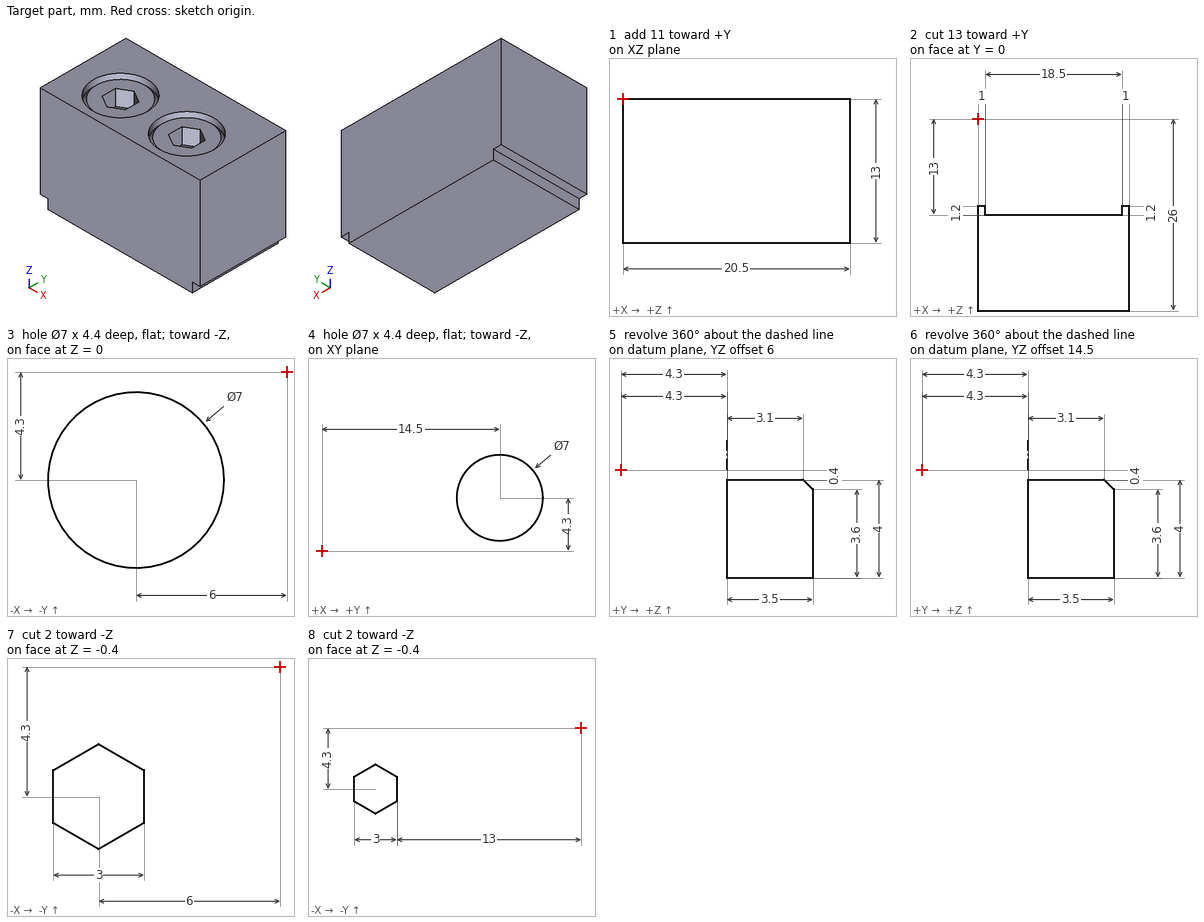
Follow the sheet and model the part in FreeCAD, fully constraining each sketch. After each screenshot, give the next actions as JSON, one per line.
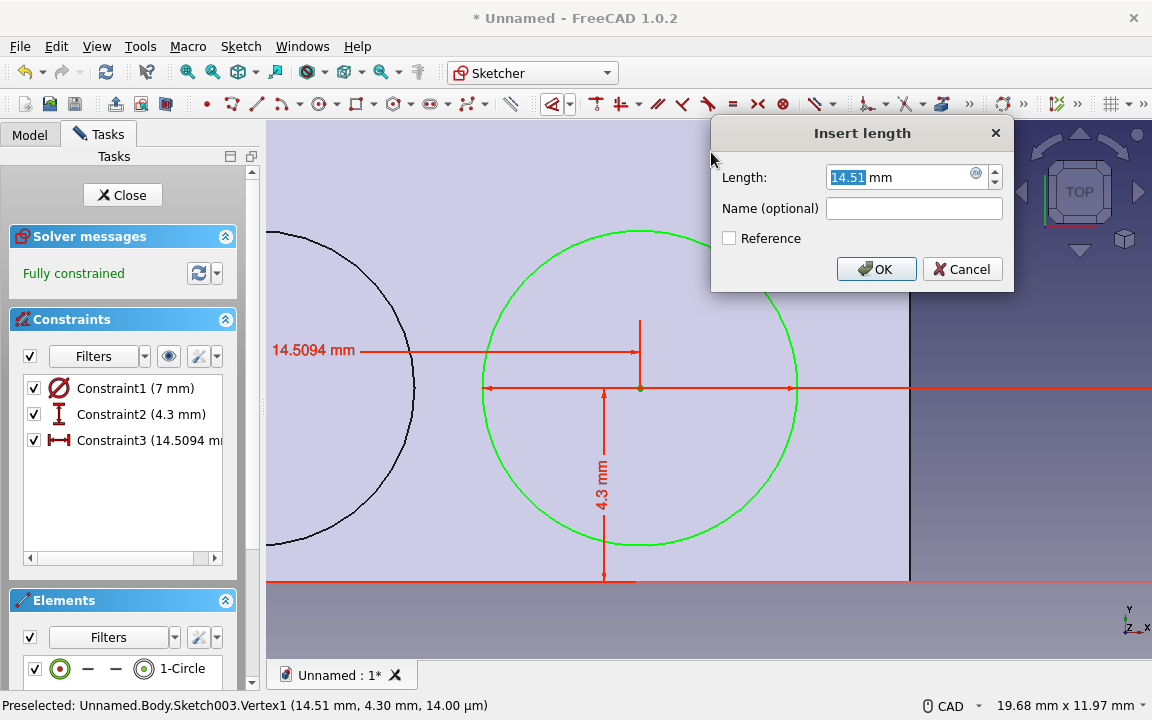
{"action": "type", "text": "14.5"}
{"action": "key", "text": "Return"}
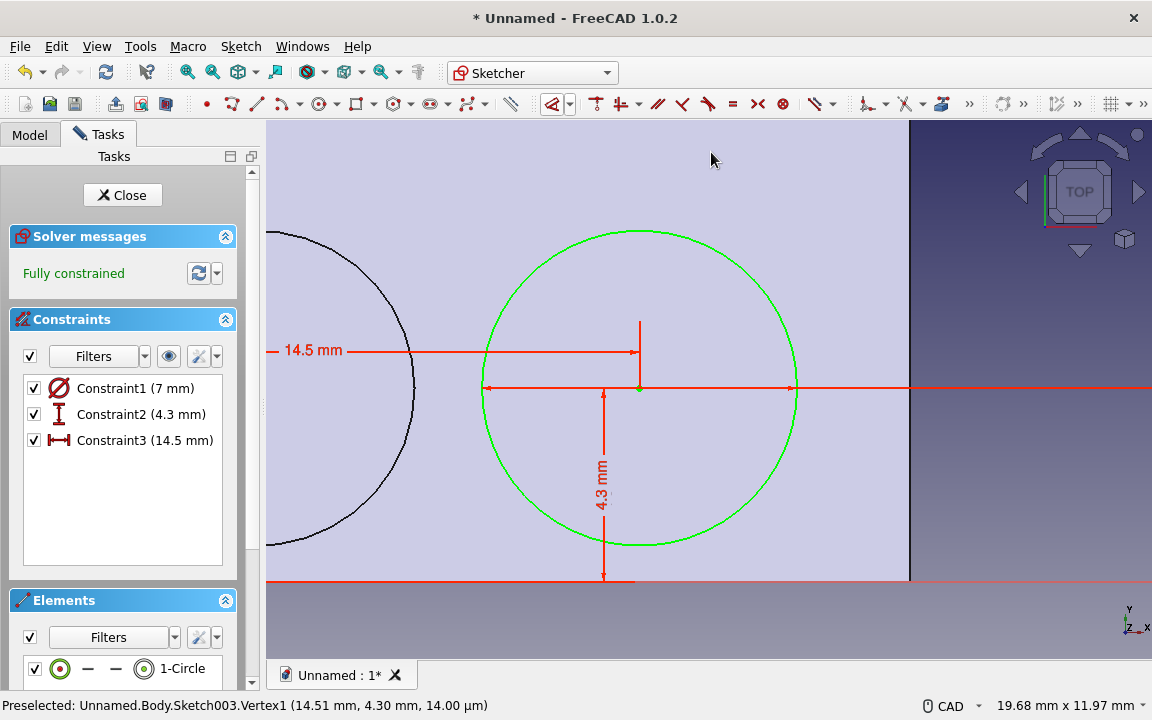
{"action": "left_click", "coordinate": [123, 195]}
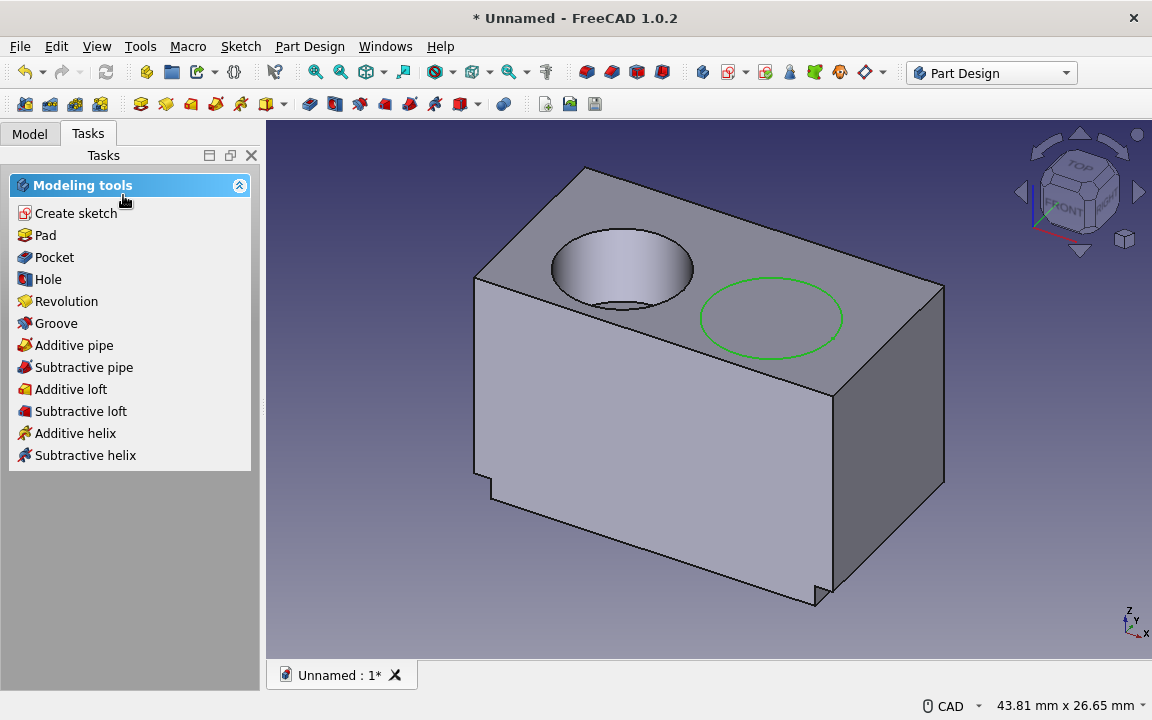
{"action": "left_click", "coordinate": [335, 104]}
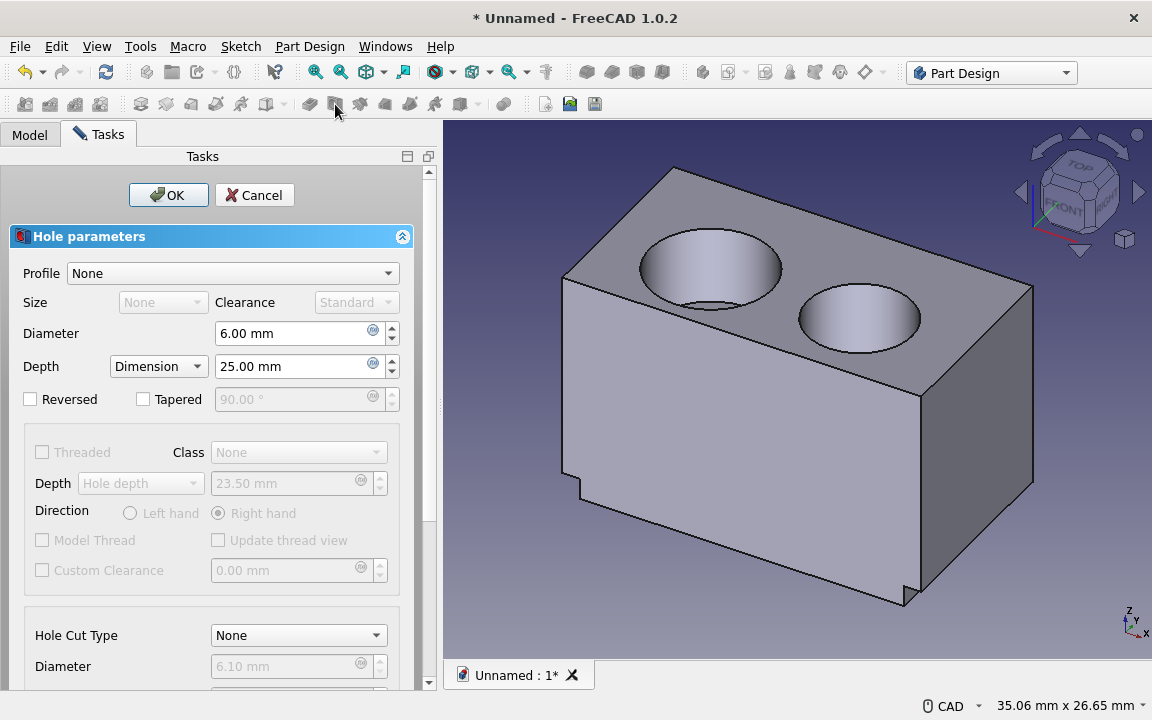
{"action": "triple_click", "coordinate": [300, 334]}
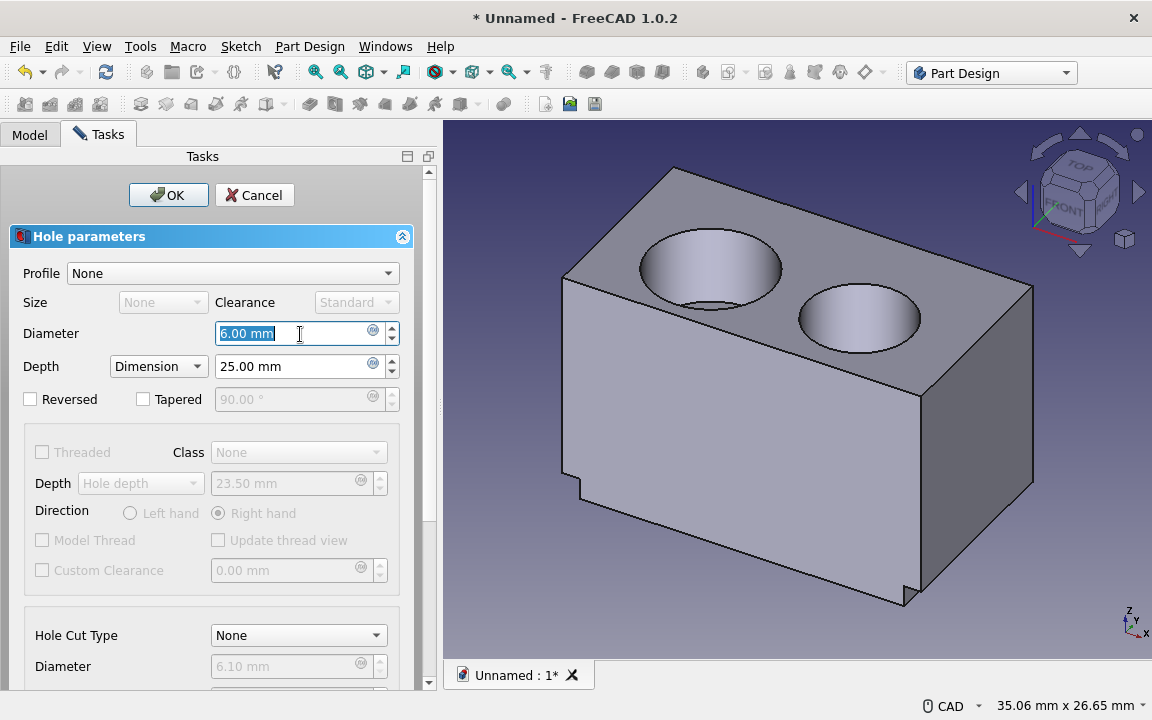
{"action": "type", "text": "7"}
{"action": "key", "text": "Tab"}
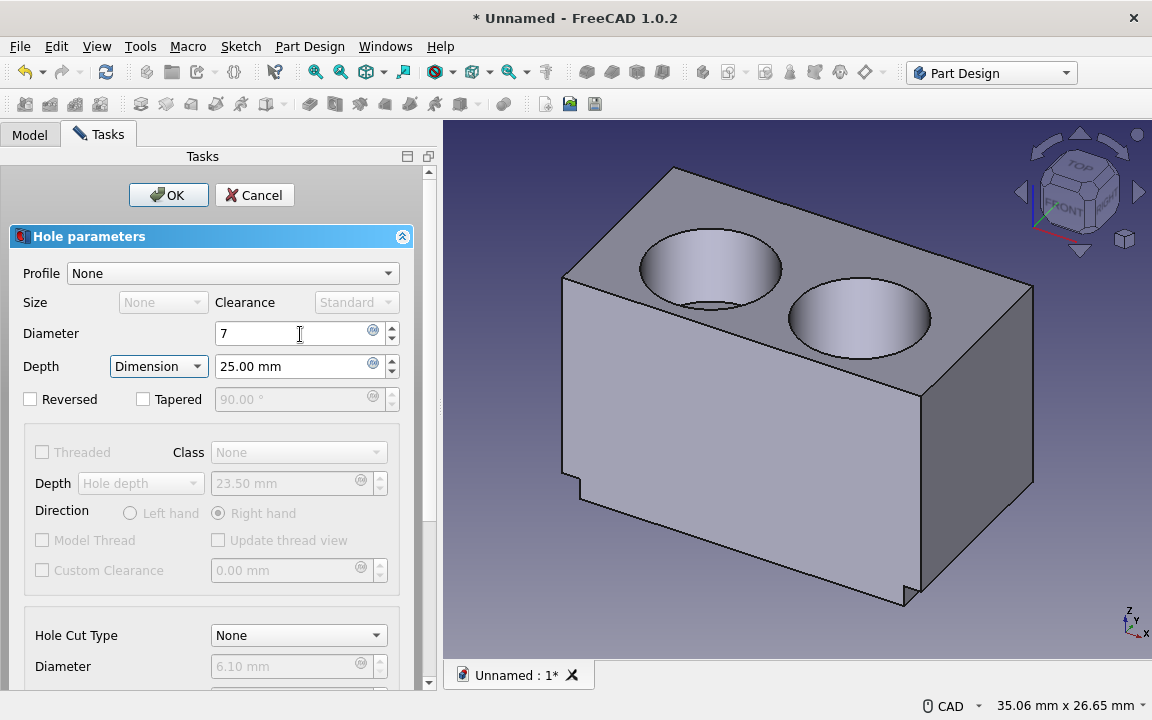
{"action": "triple_click", "coordinate": [300, 366]}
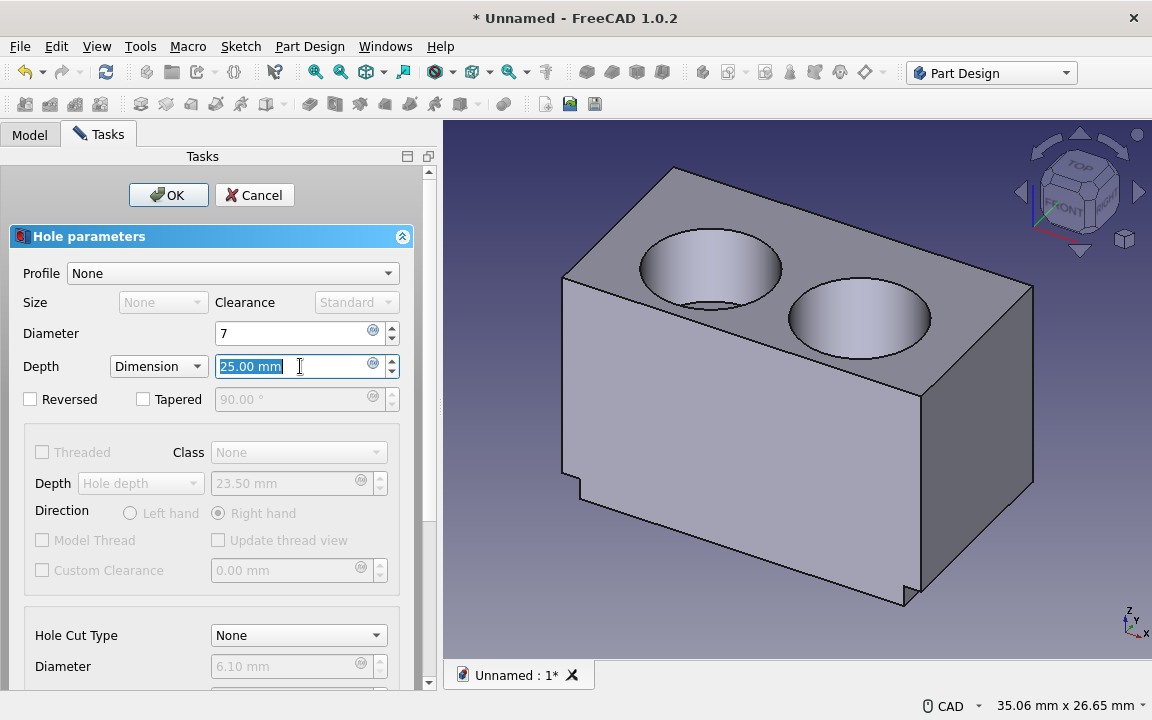
{"action": "type", "text": "4.4"}
{"action": "key", "text": "Tab"}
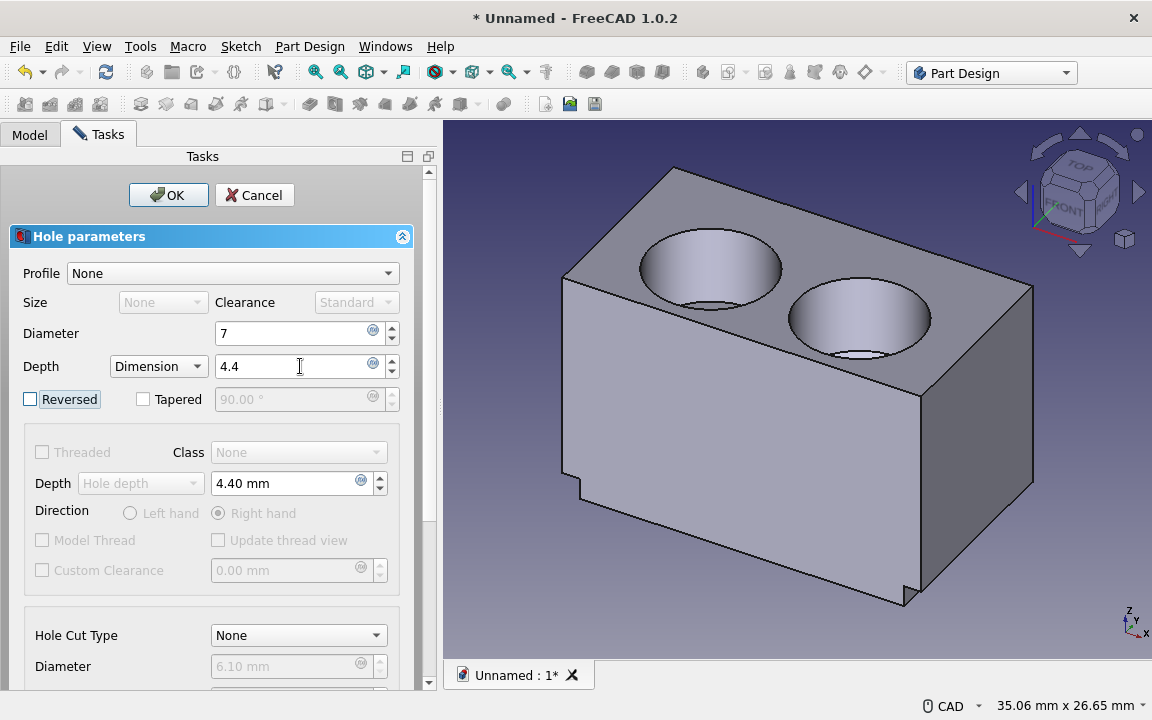
{"action": "scroll", "coordinate": [429, 428], "scroll_direction": "down", "scroll_amount": 4}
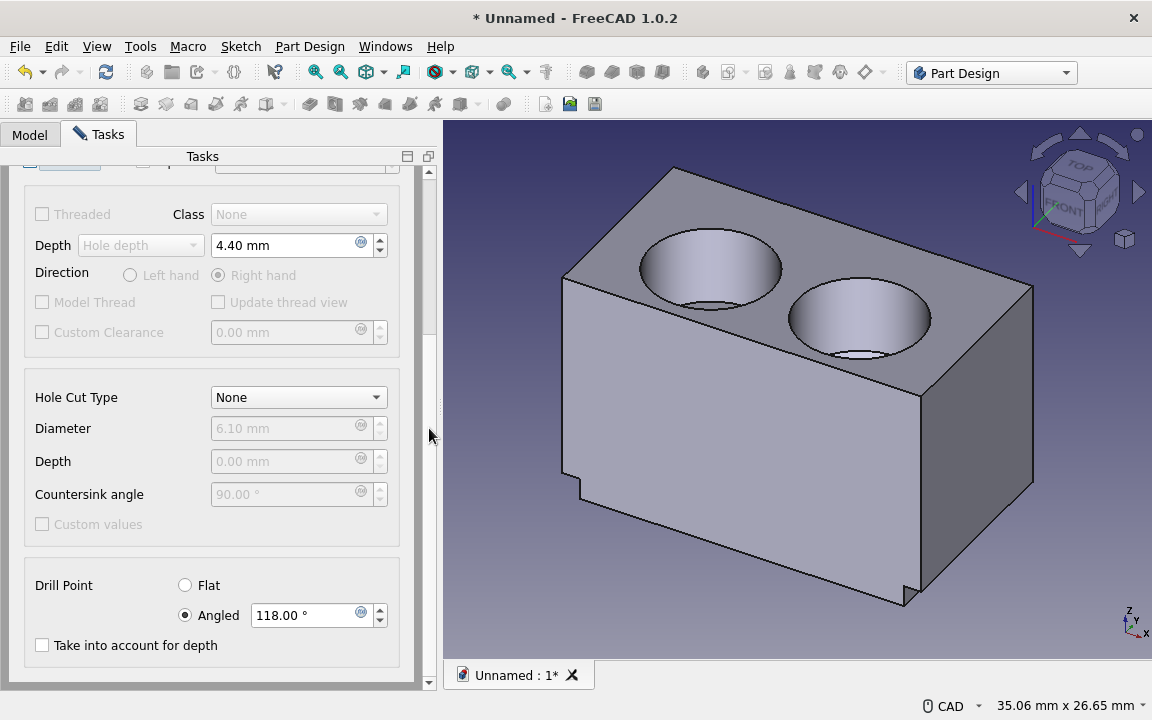
{"action": "left_click", "coordinate": [186, 583]}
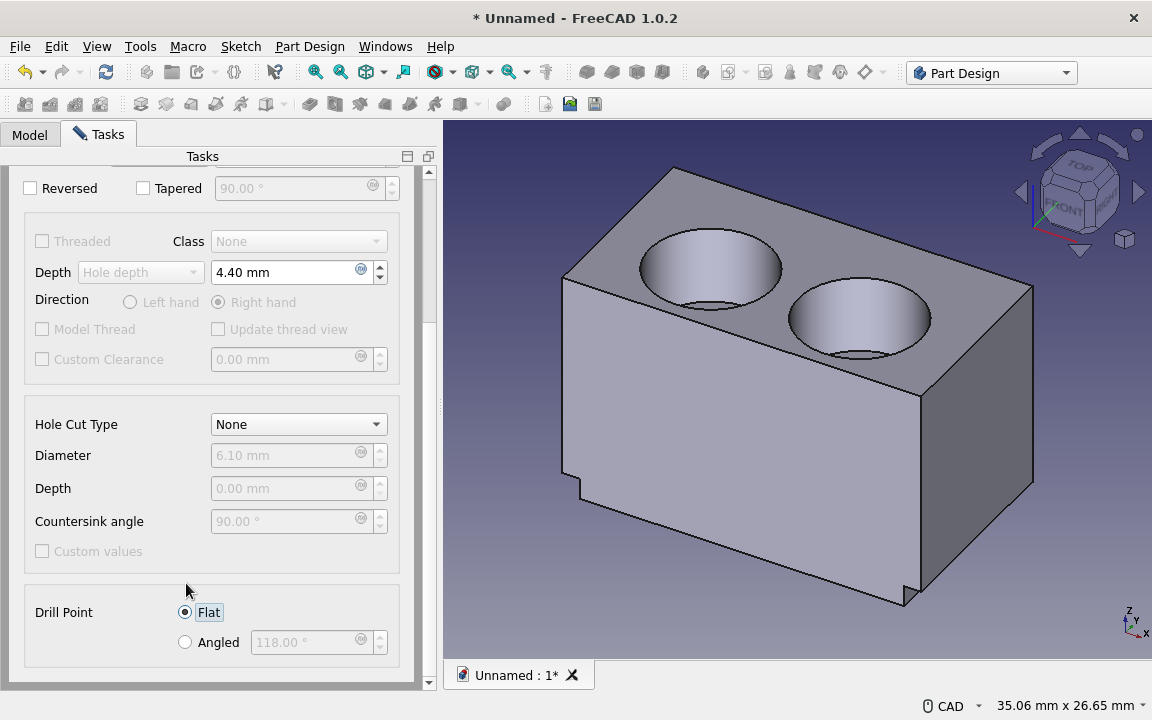
{"action": "scroll", "coordinate": [429, 428], "scroll_direction": "up", "scroll_amount": 5}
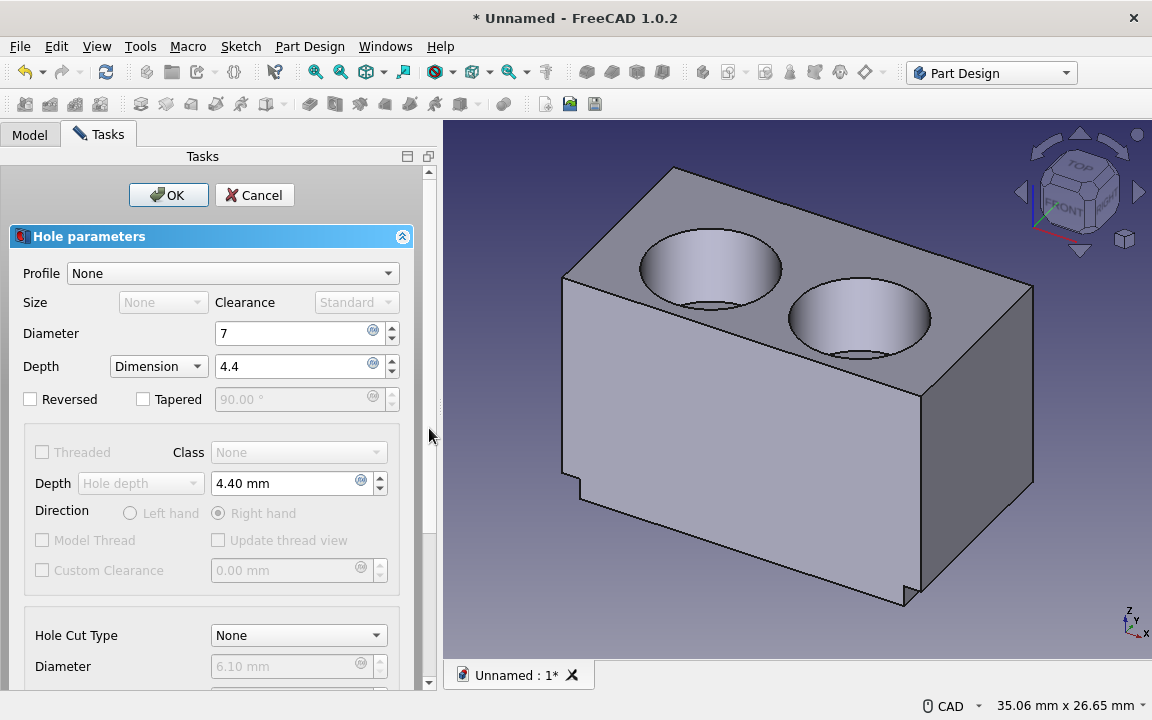
{"action": "left_click", "coordinate": [169, 195]}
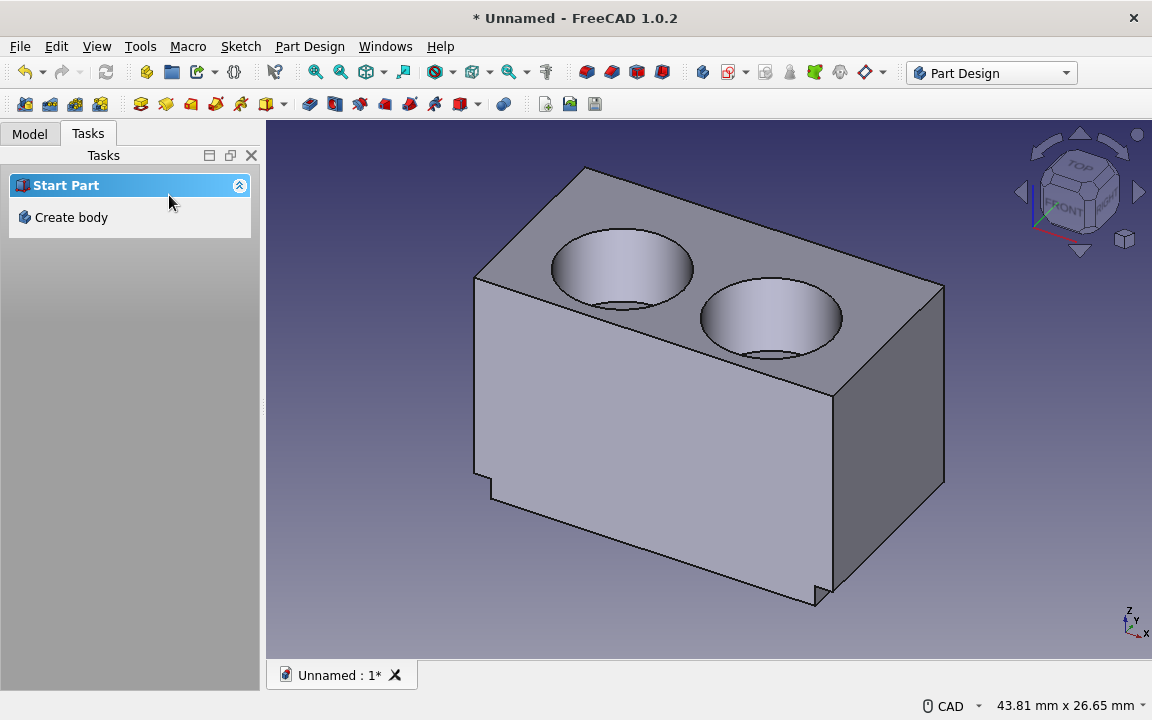
{"action": "left_click", "coordinate": [30, 134]}